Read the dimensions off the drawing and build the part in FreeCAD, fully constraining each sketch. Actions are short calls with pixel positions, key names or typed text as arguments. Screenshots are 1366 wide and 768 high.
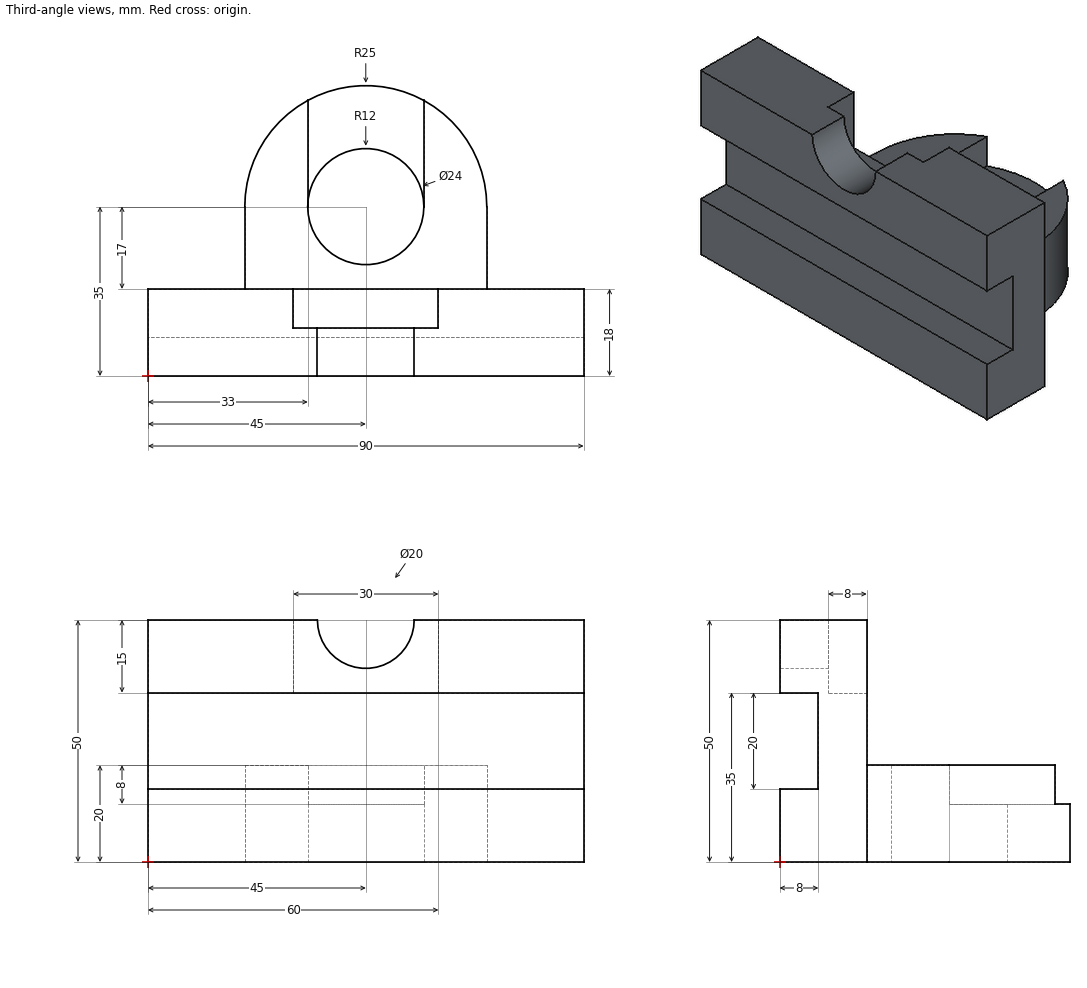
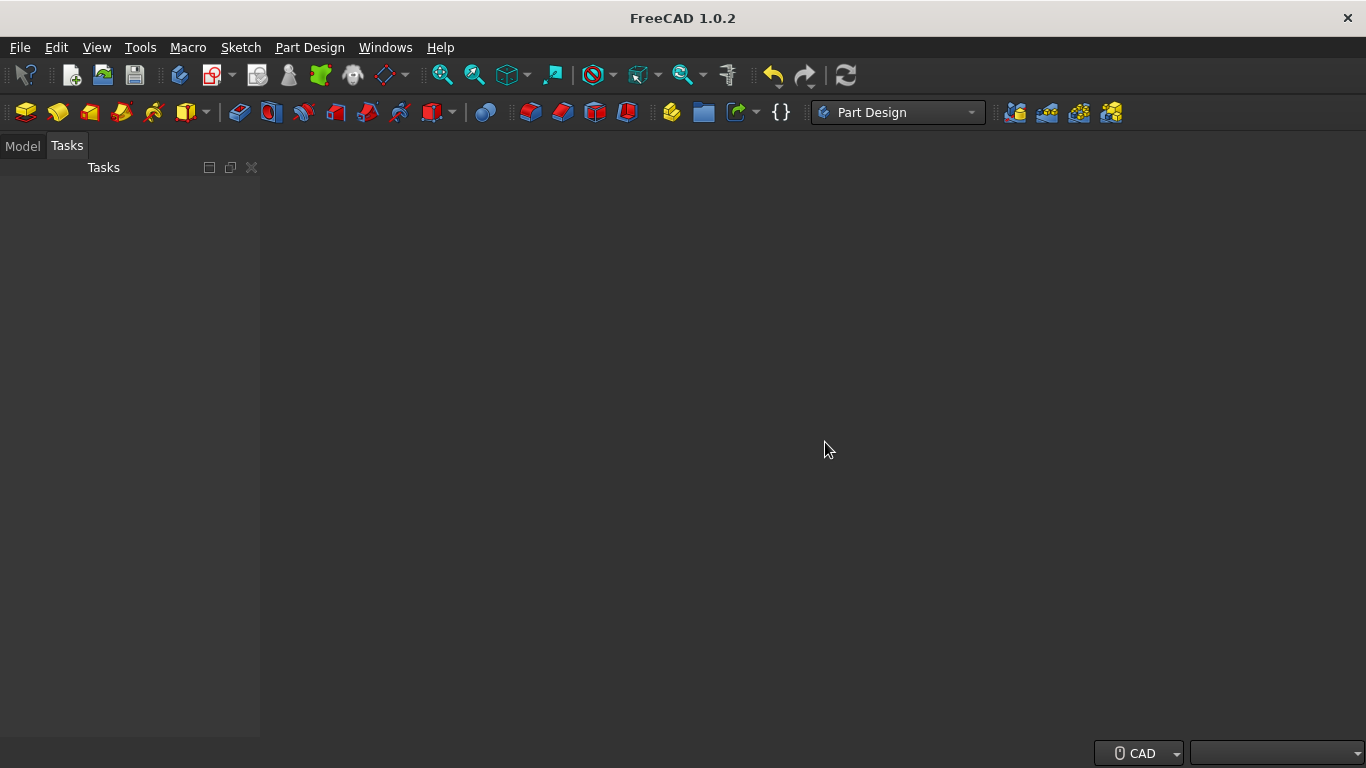
key(ctrl+n)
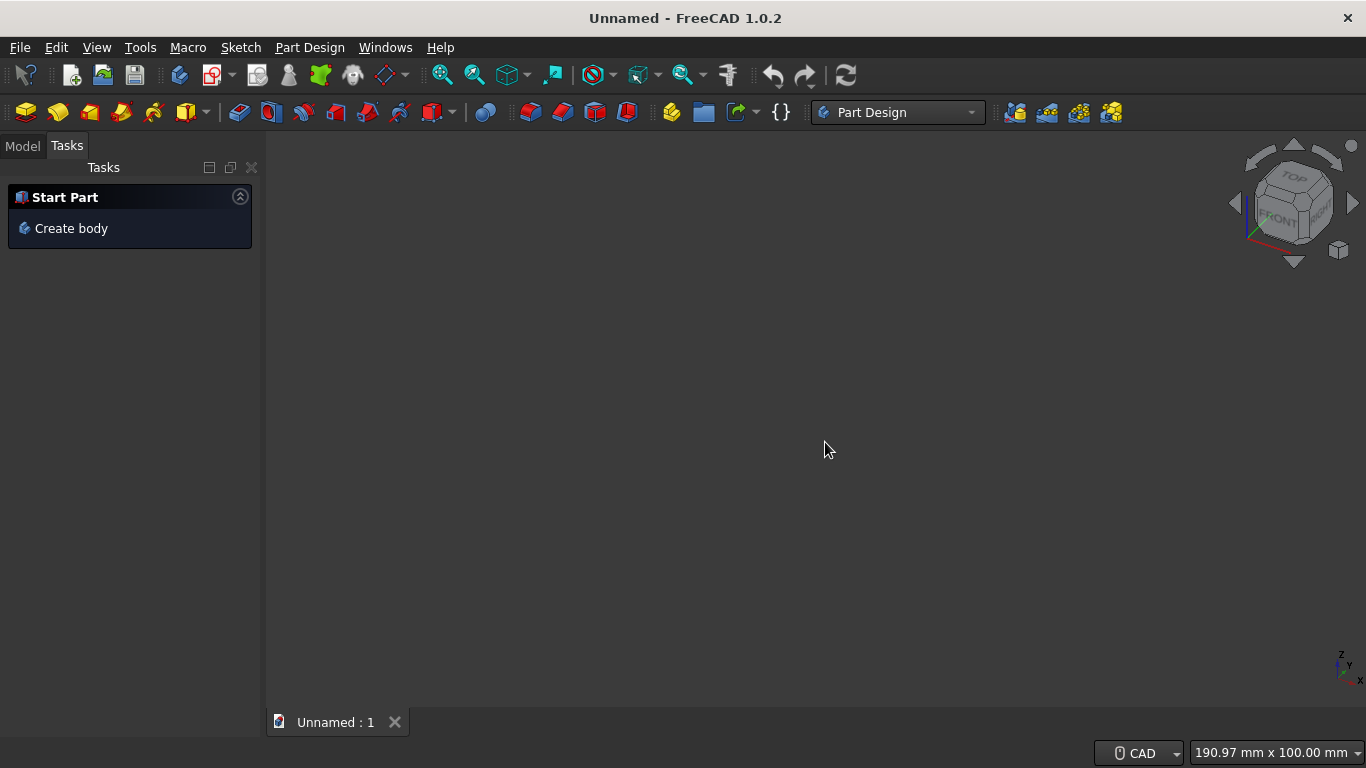
click(212, 76)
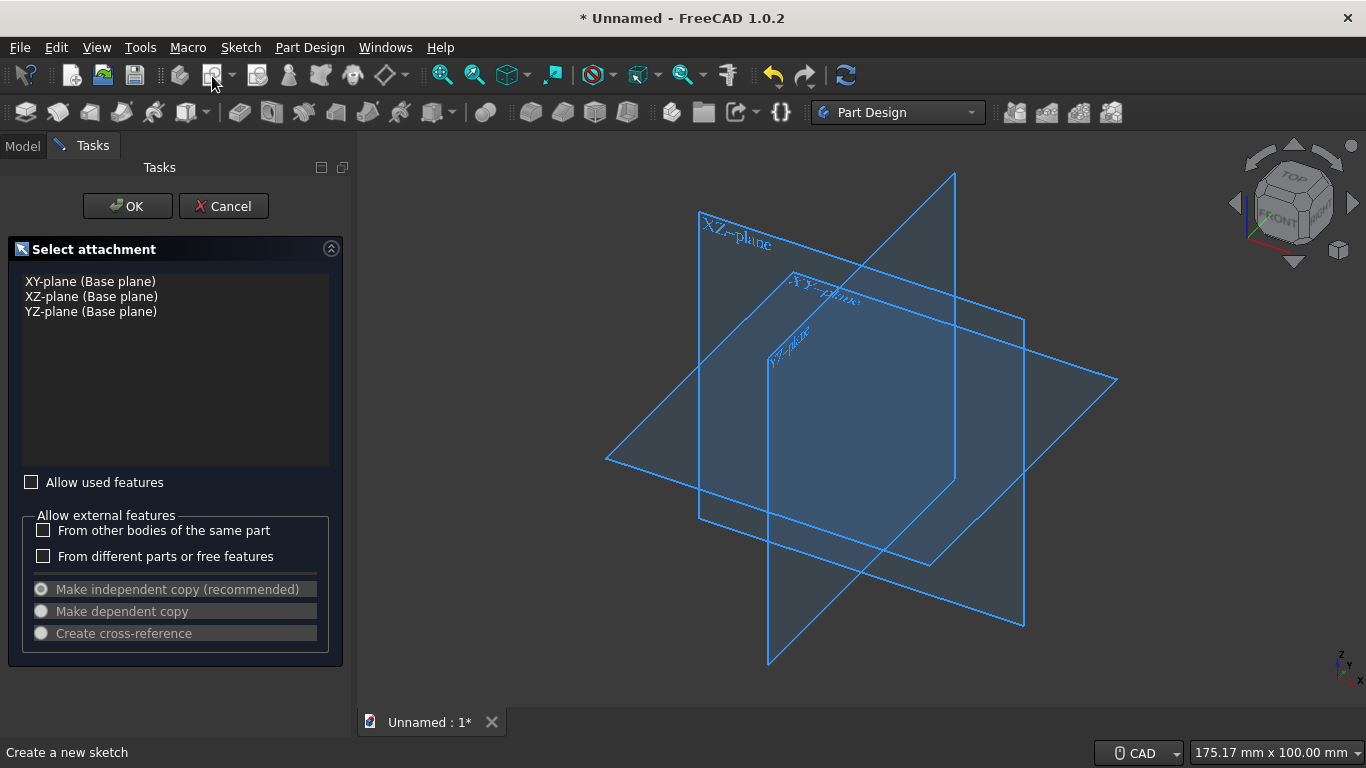
click(82, 282)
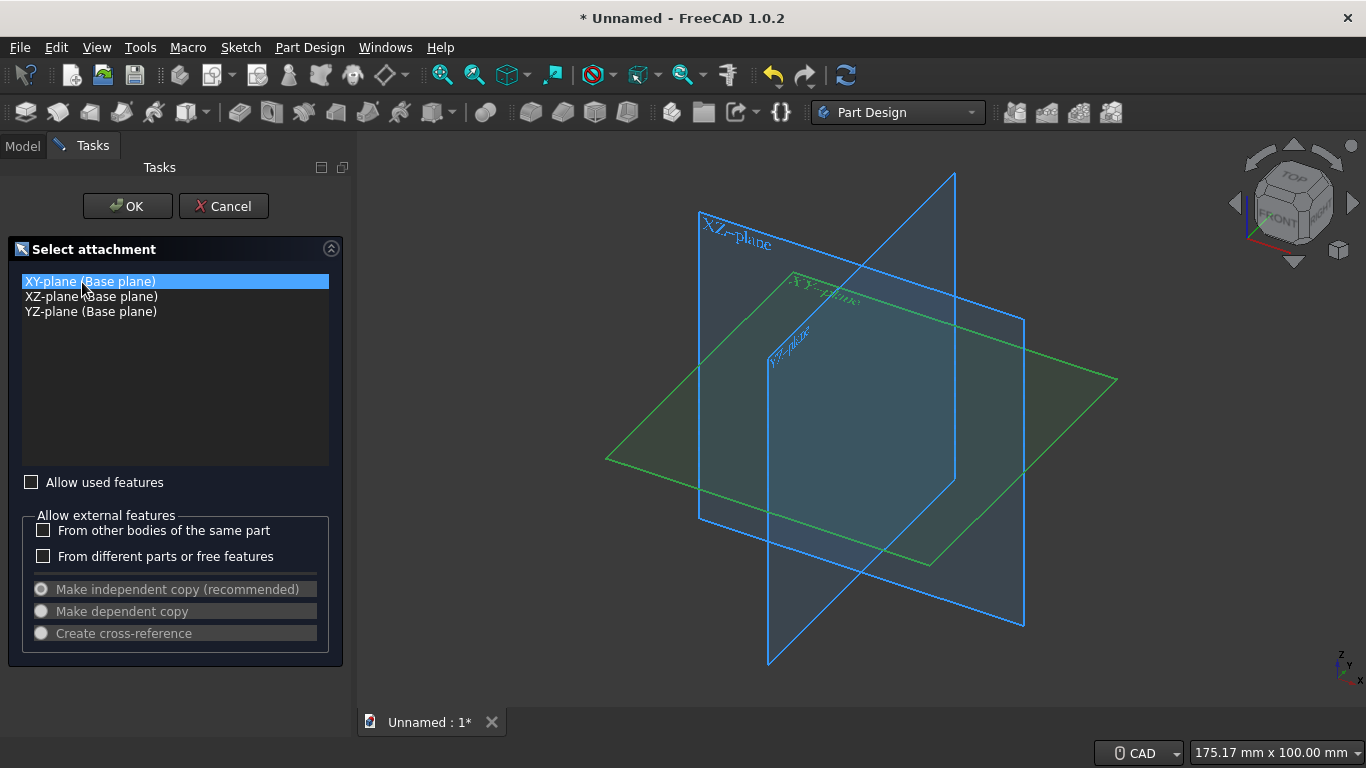
click(128, 206)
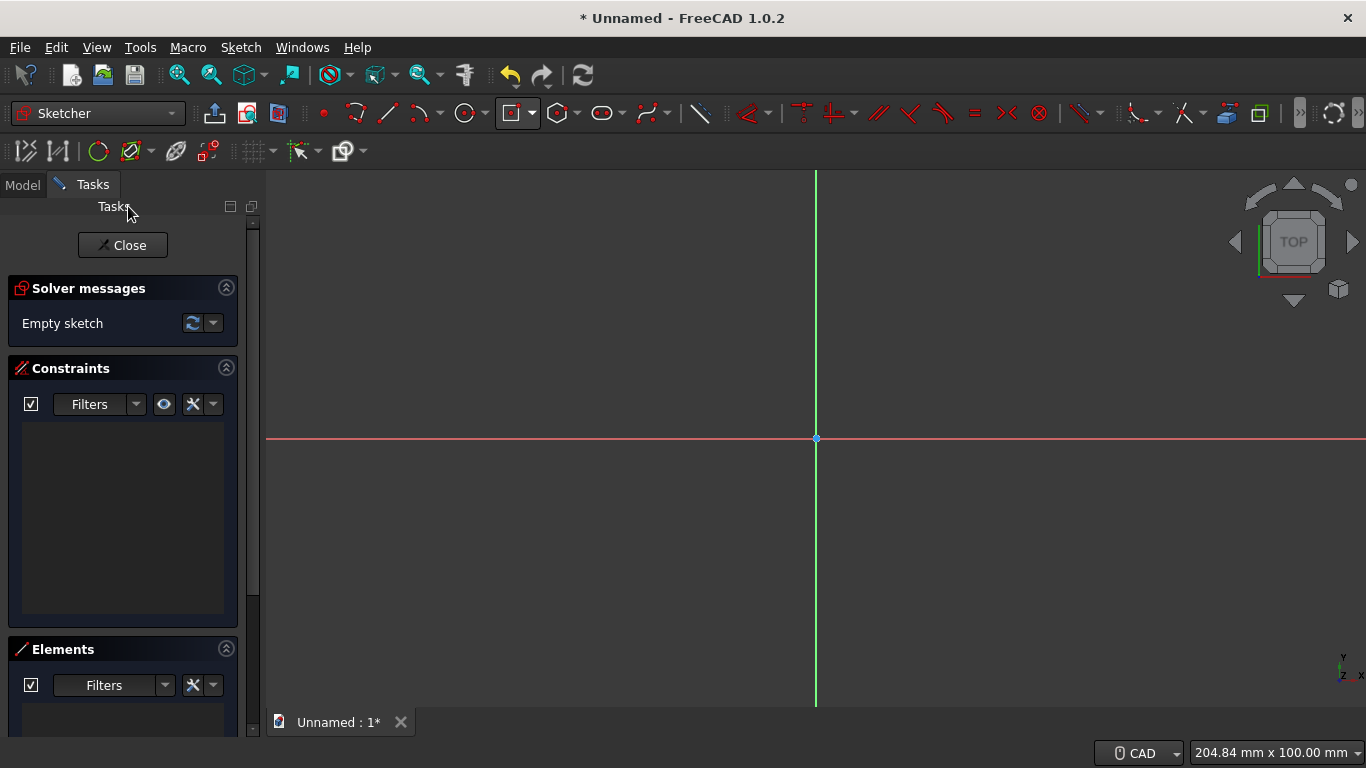
scroll(294, 657, down, 1)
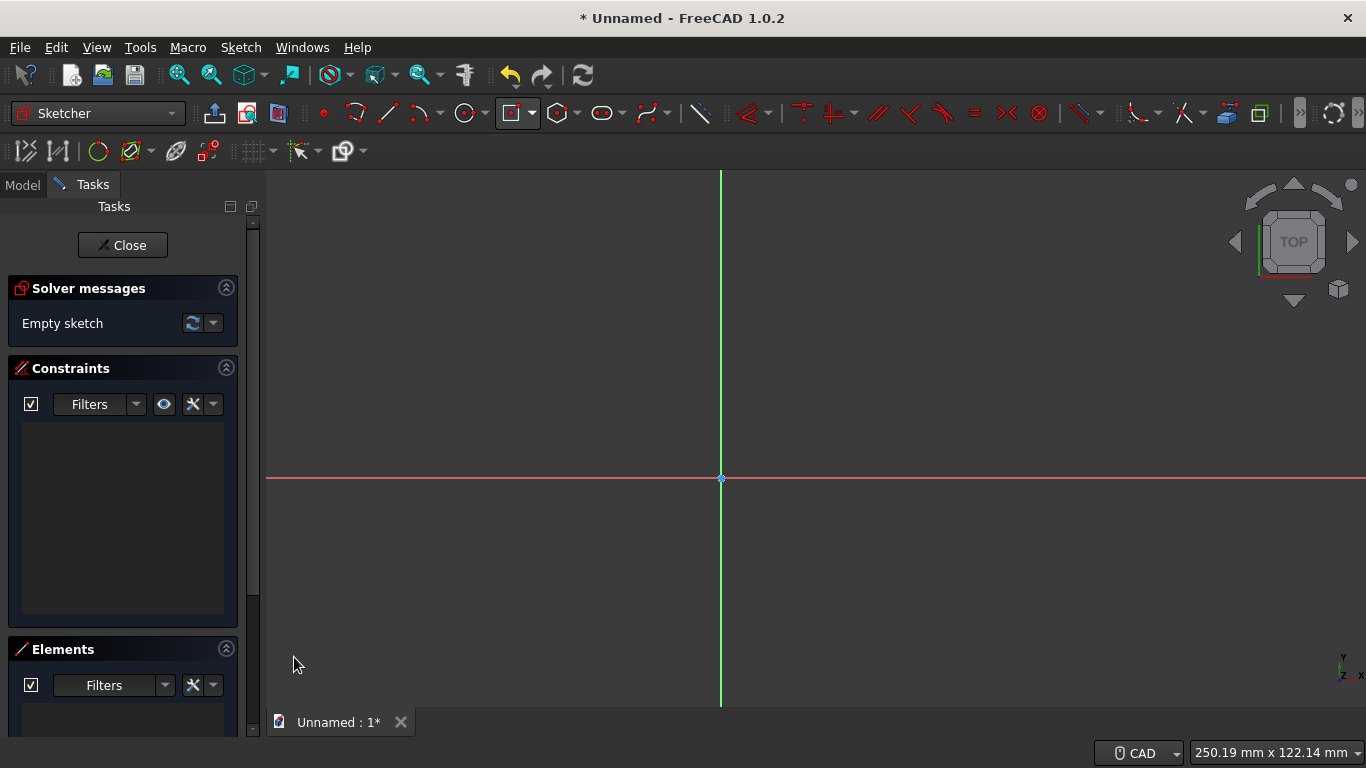
scroll(1201, 439, up, 2)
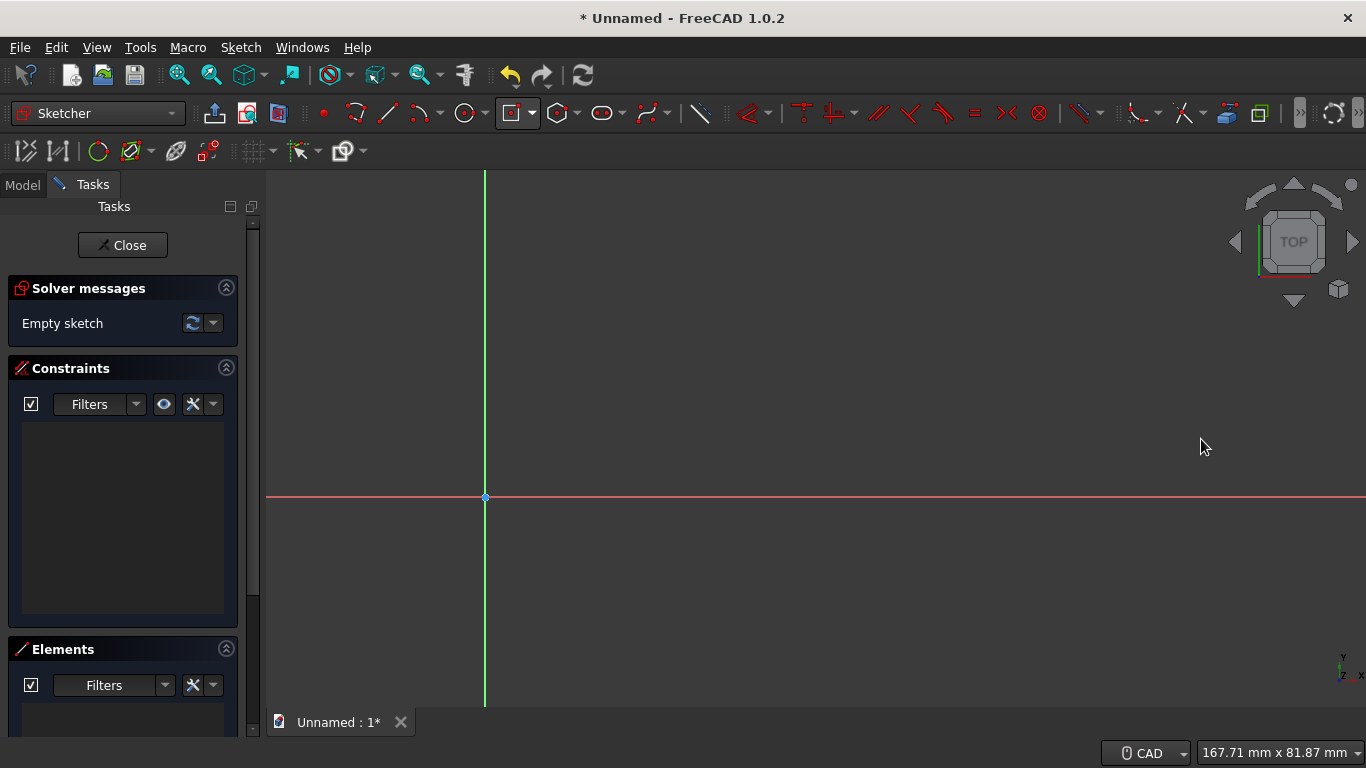
click(534, 114)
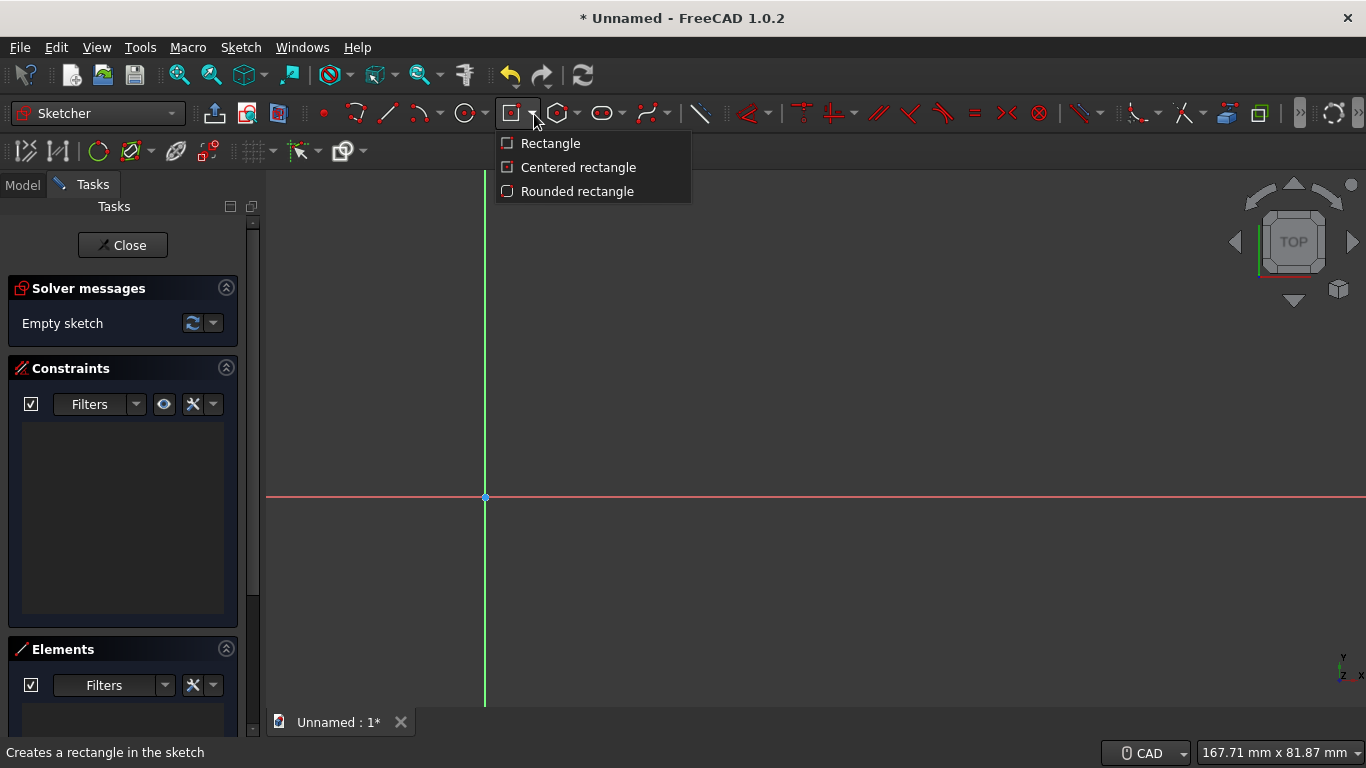
click(594, 143)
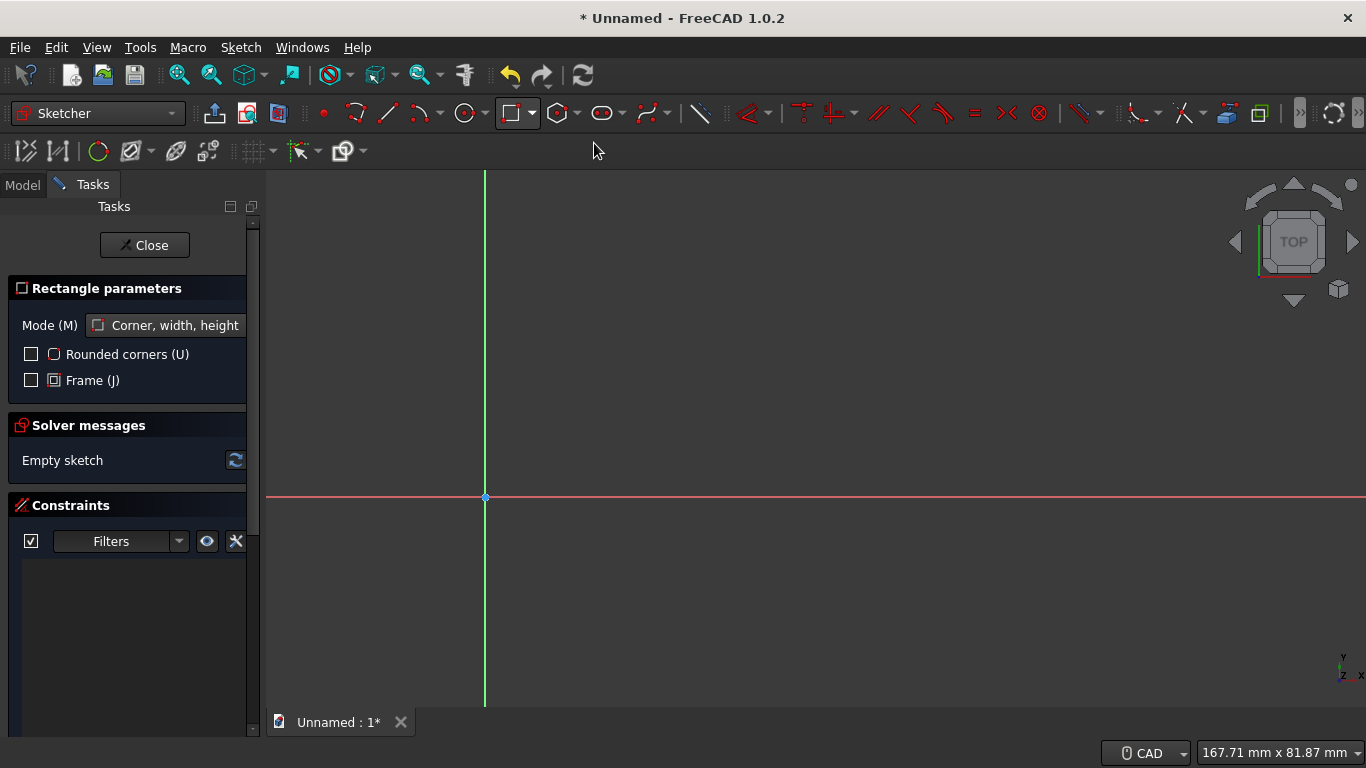
click(485, 497)
move(1075, 379)